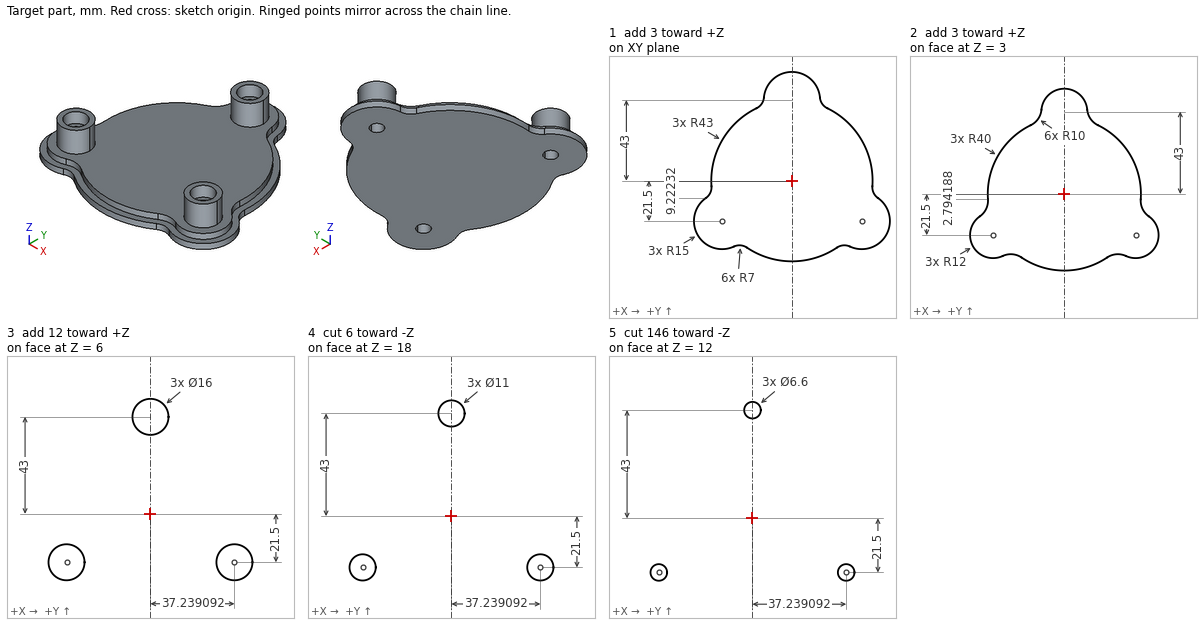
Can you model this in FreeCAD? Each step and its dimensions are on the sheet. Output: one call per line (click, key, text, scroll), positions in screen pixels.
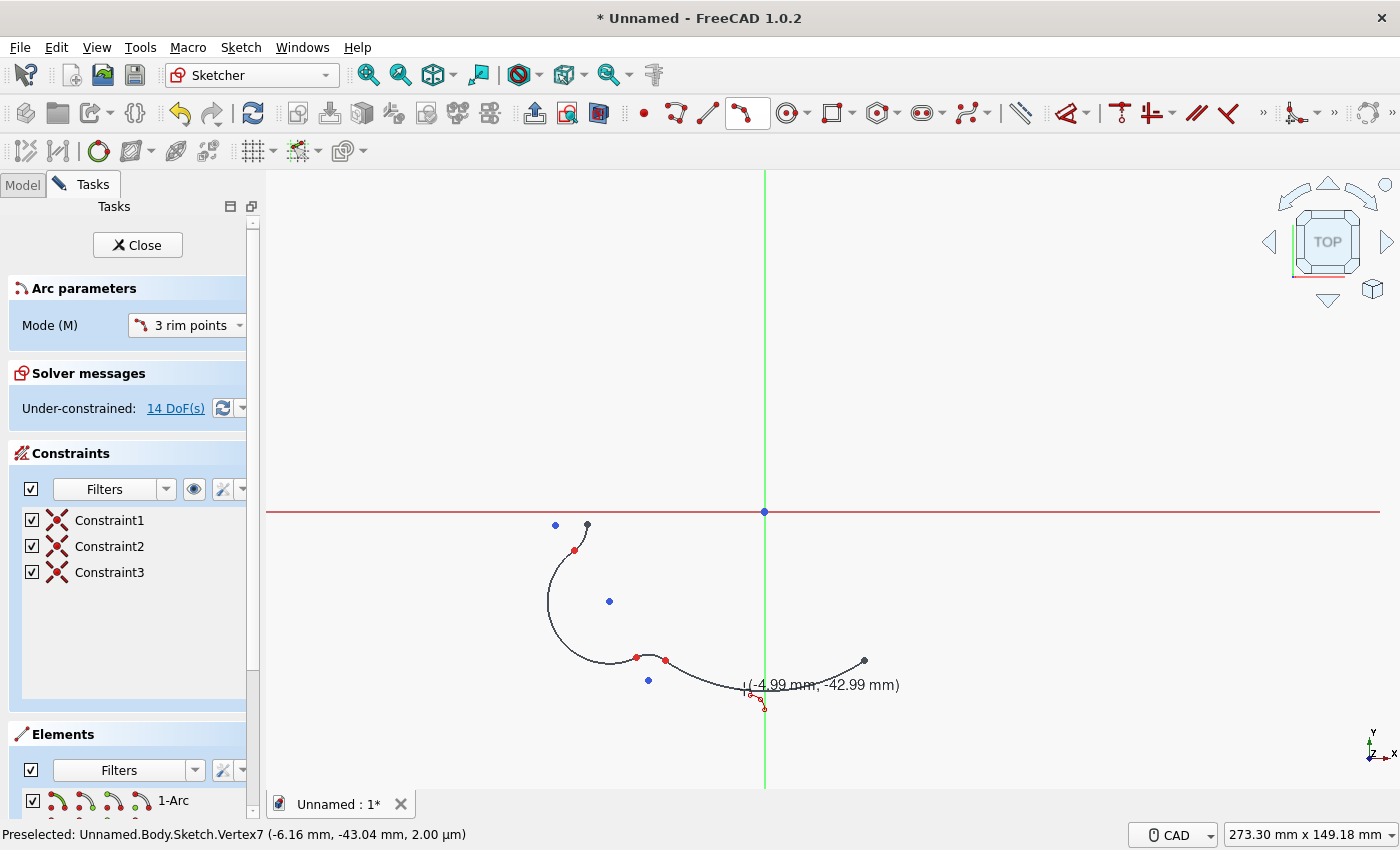
click(864, 661)
click(893, 657)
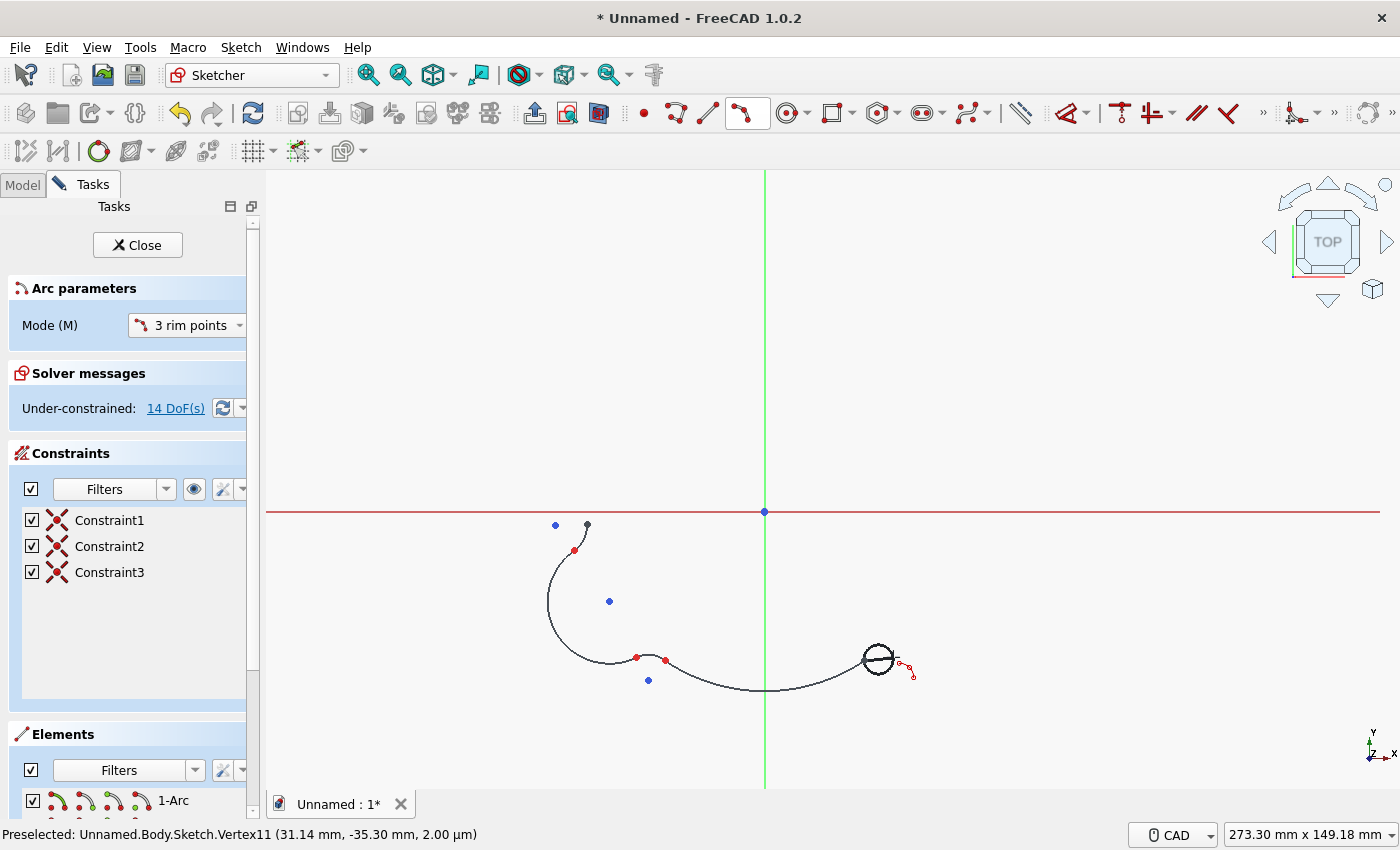
scroll(878, 655, up, 8)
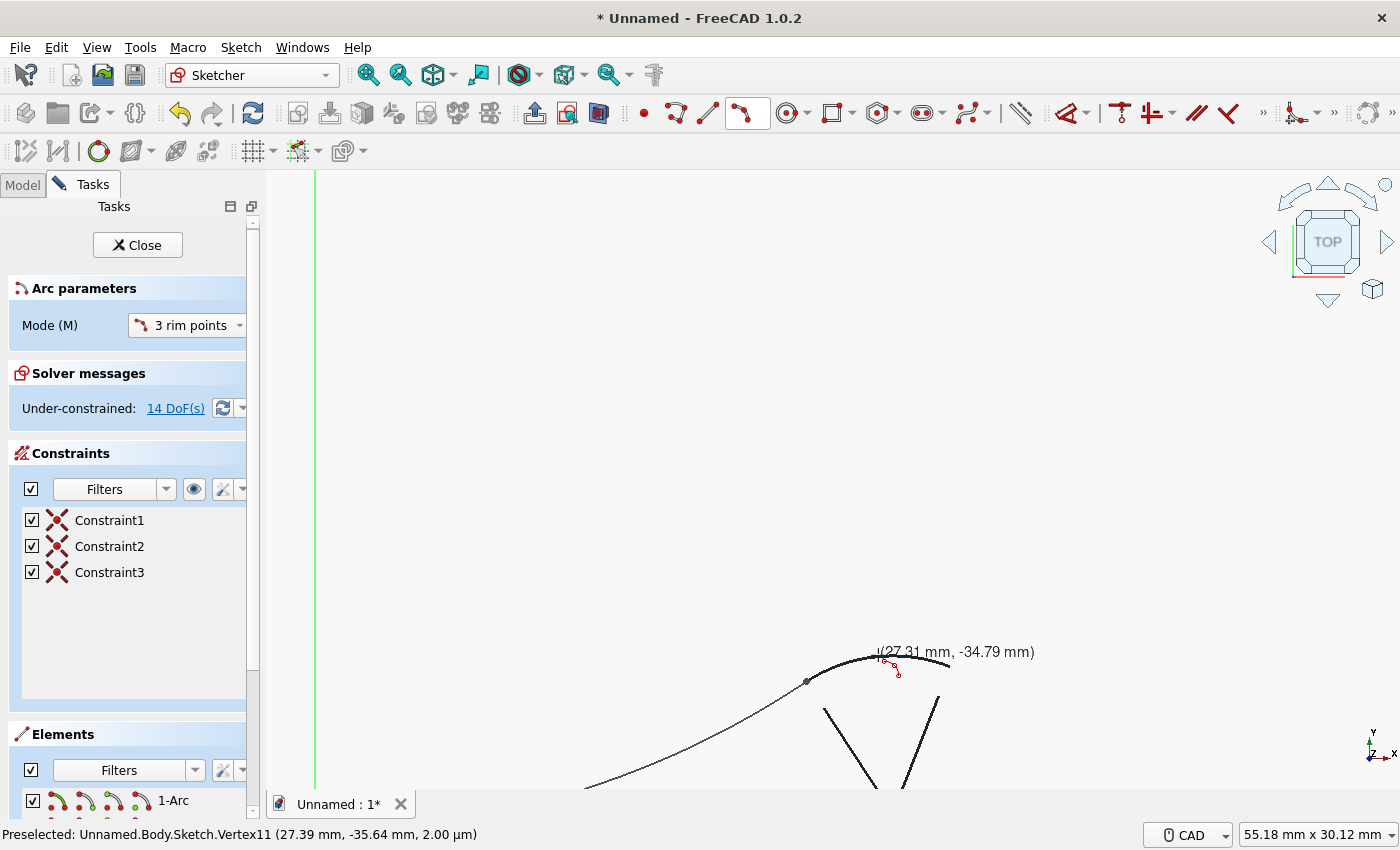
click(878, 650)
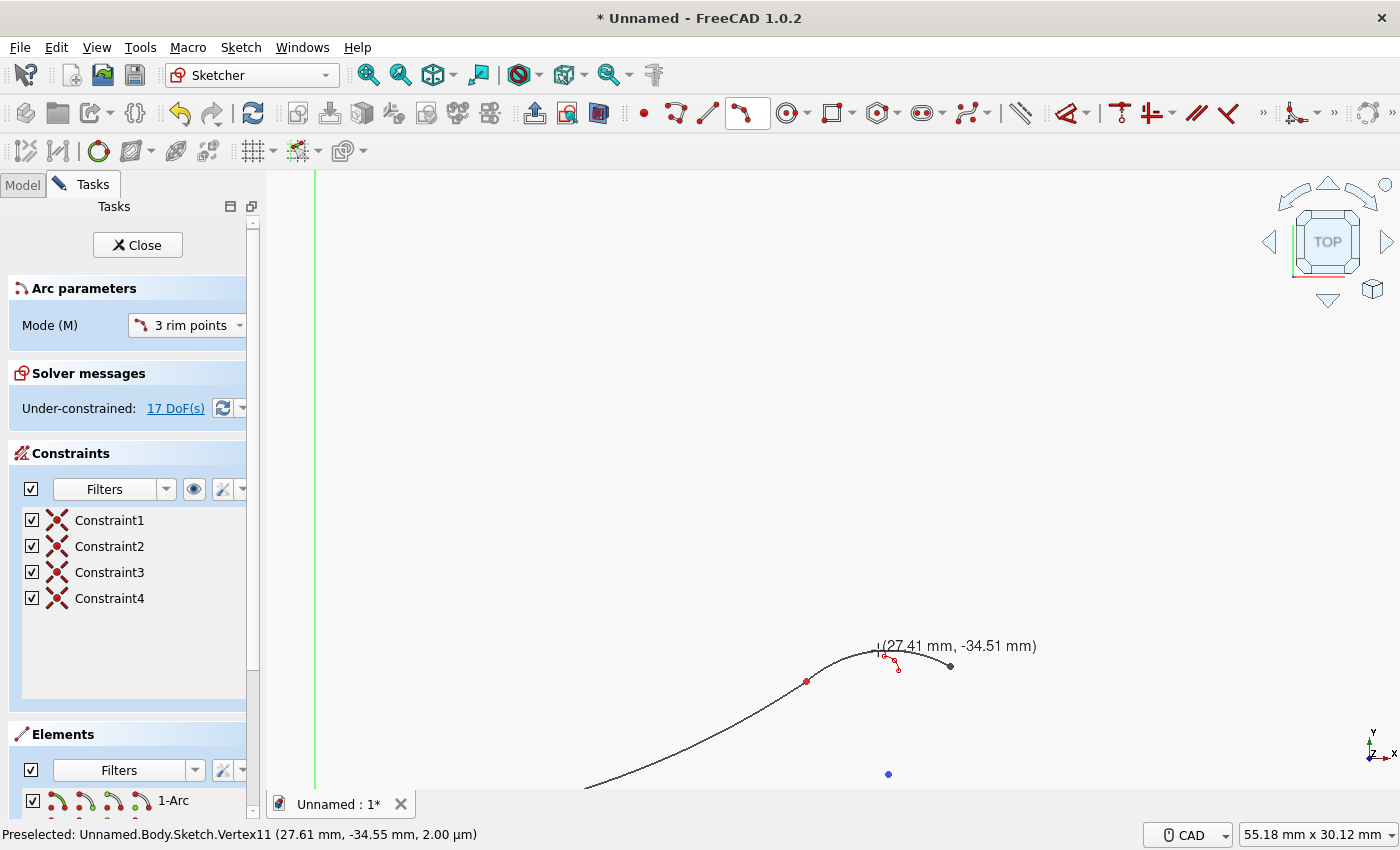
scroll(878, 655, down, 8)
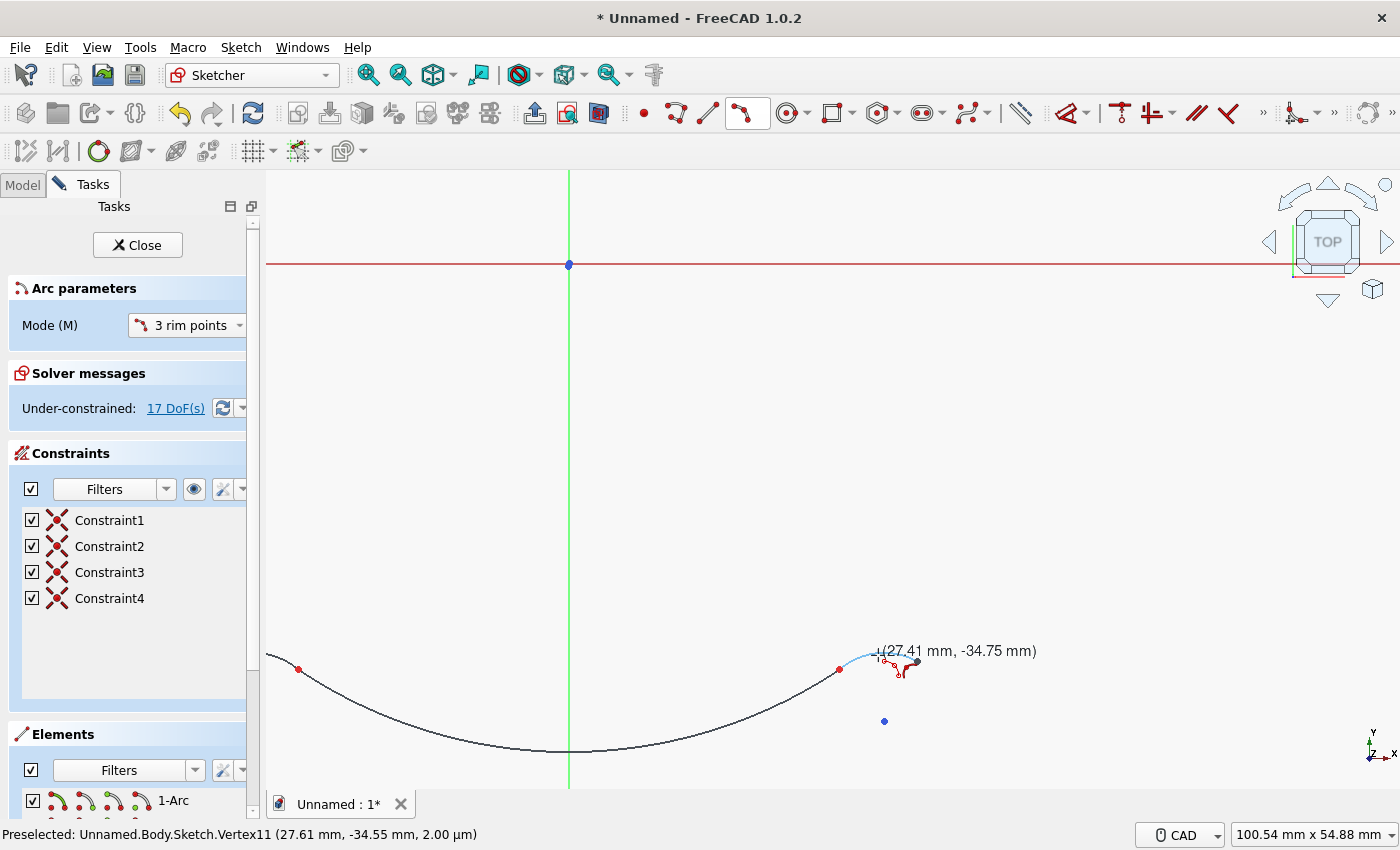
click(893, 658)
click(955, 550)
click(973, 632)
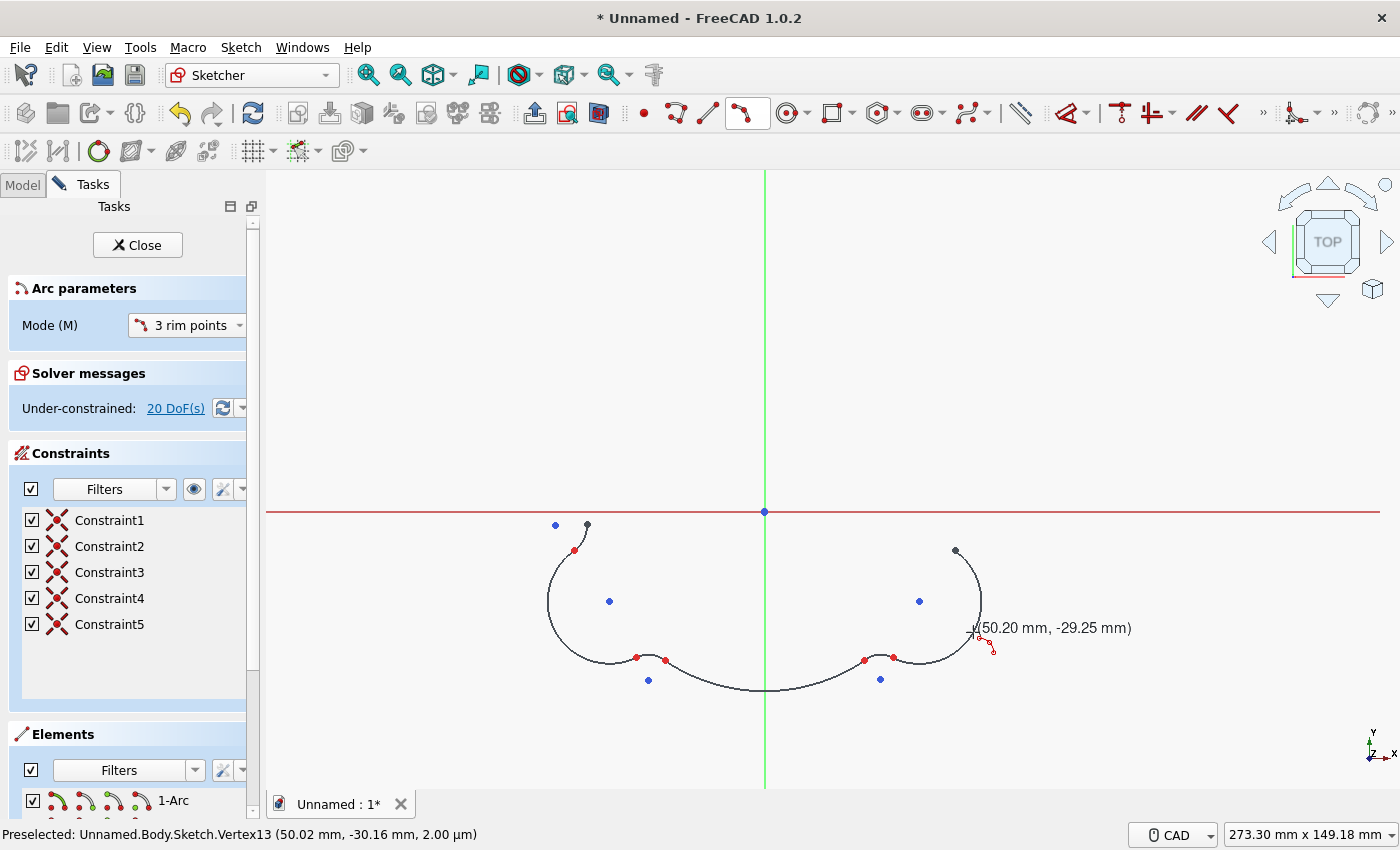
click(955, 551)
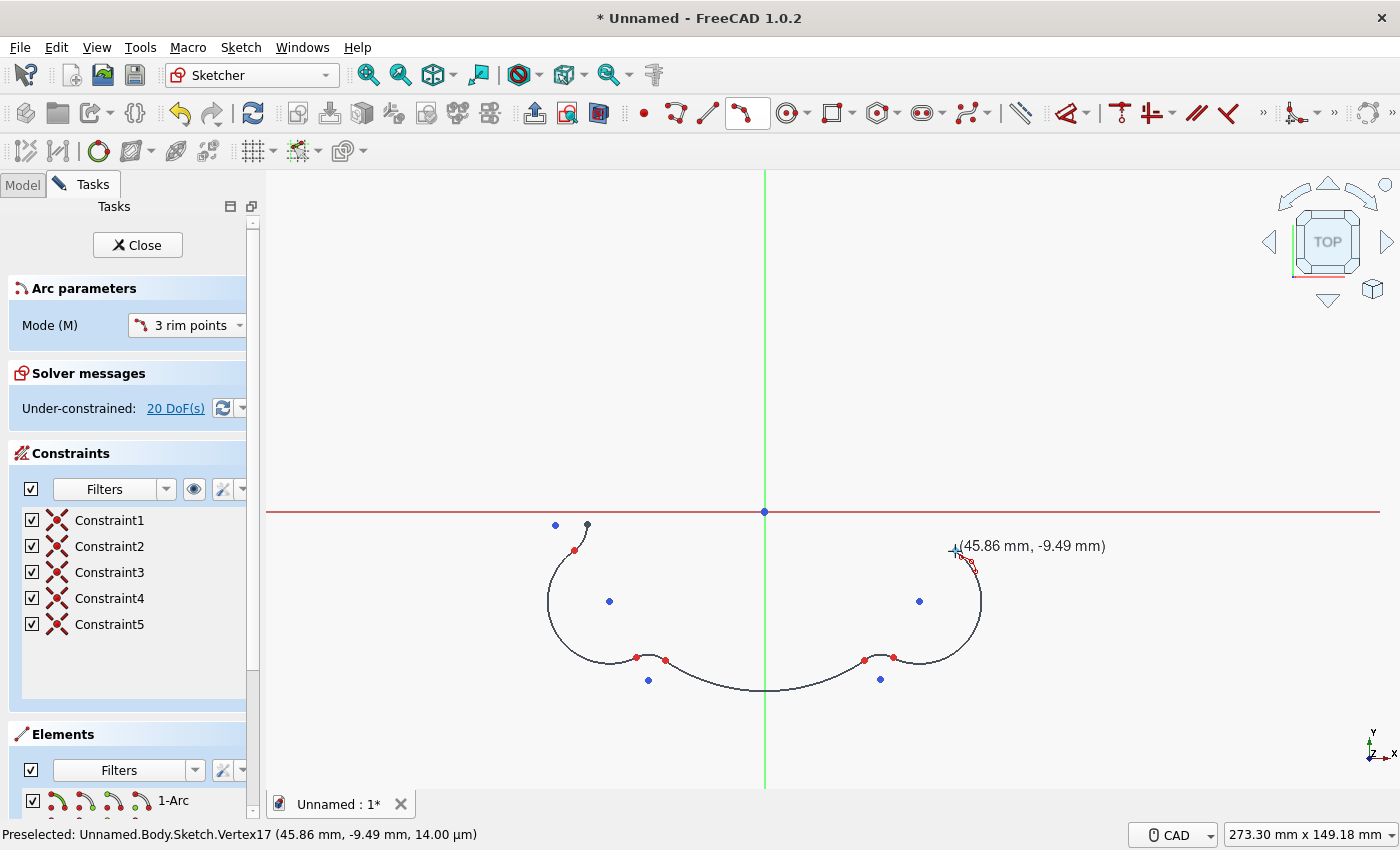
scroll(943, 524, up, 2)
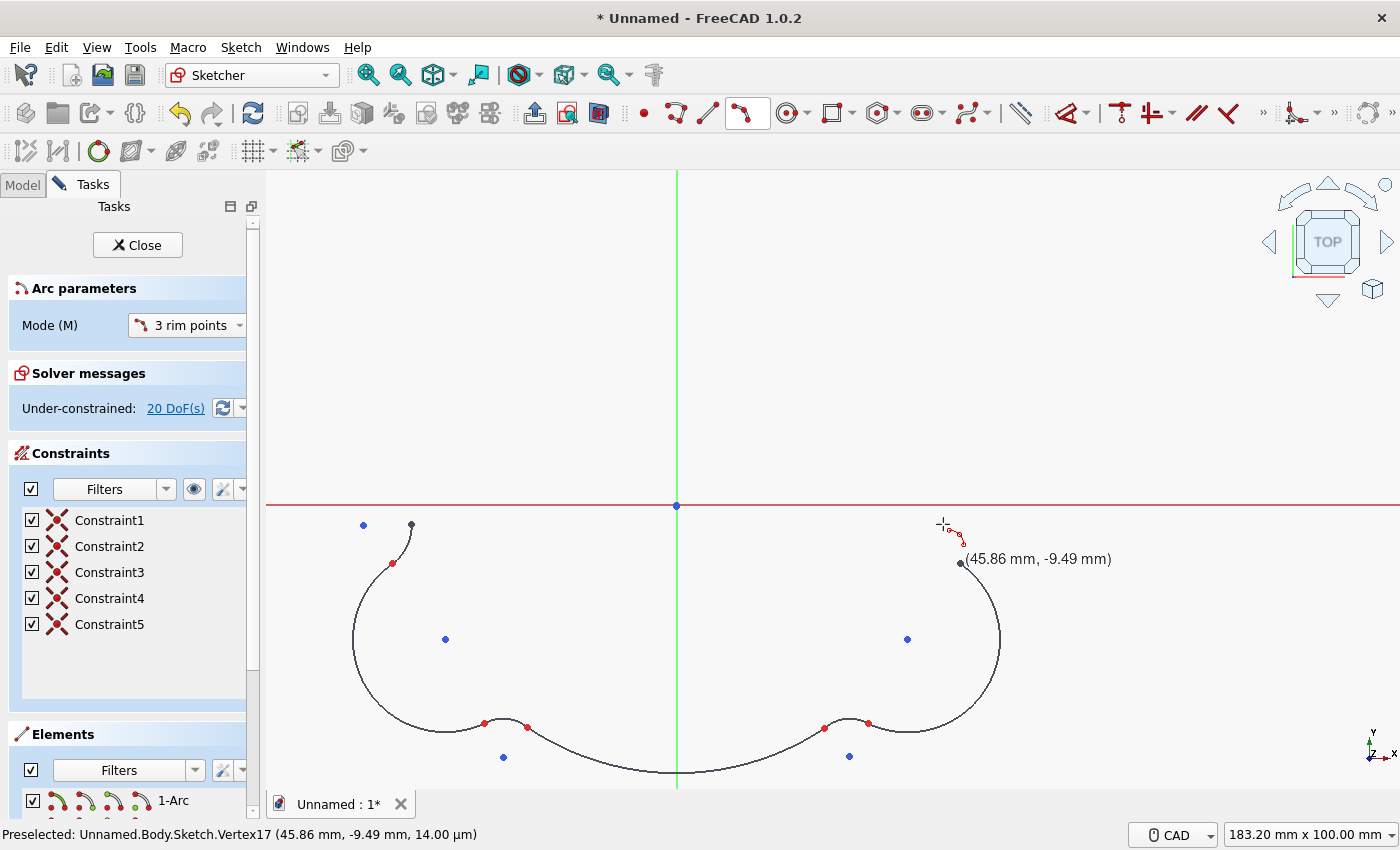
click(942, 524)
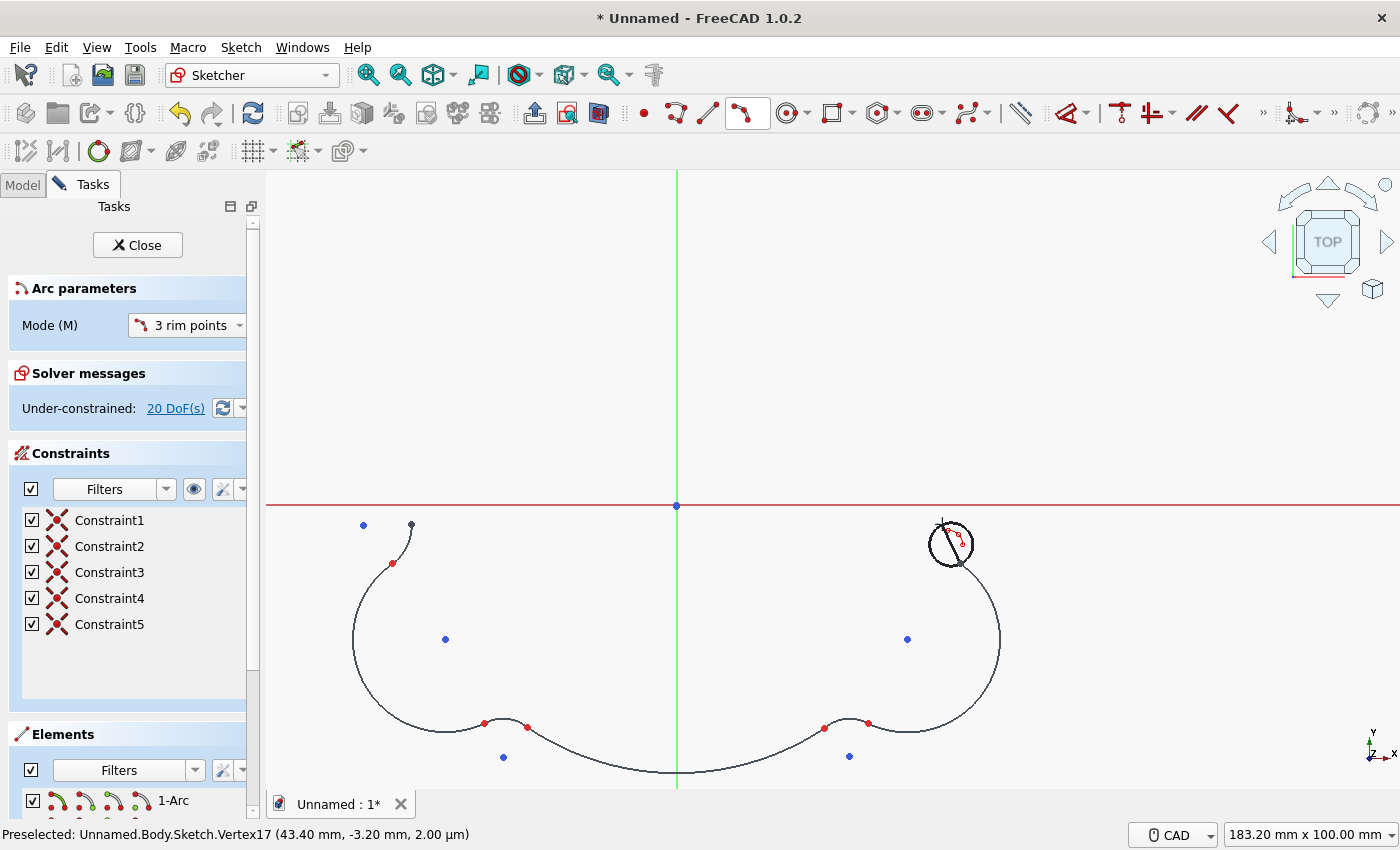
scroll(946, 546, up, 6)